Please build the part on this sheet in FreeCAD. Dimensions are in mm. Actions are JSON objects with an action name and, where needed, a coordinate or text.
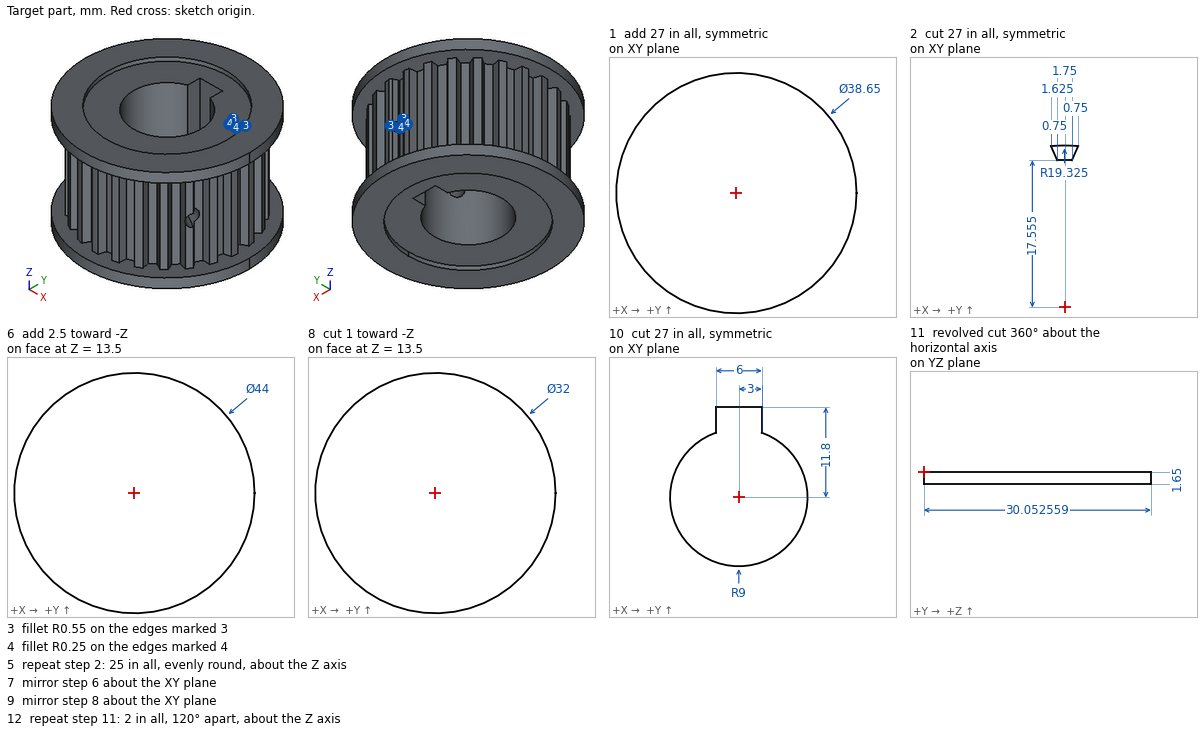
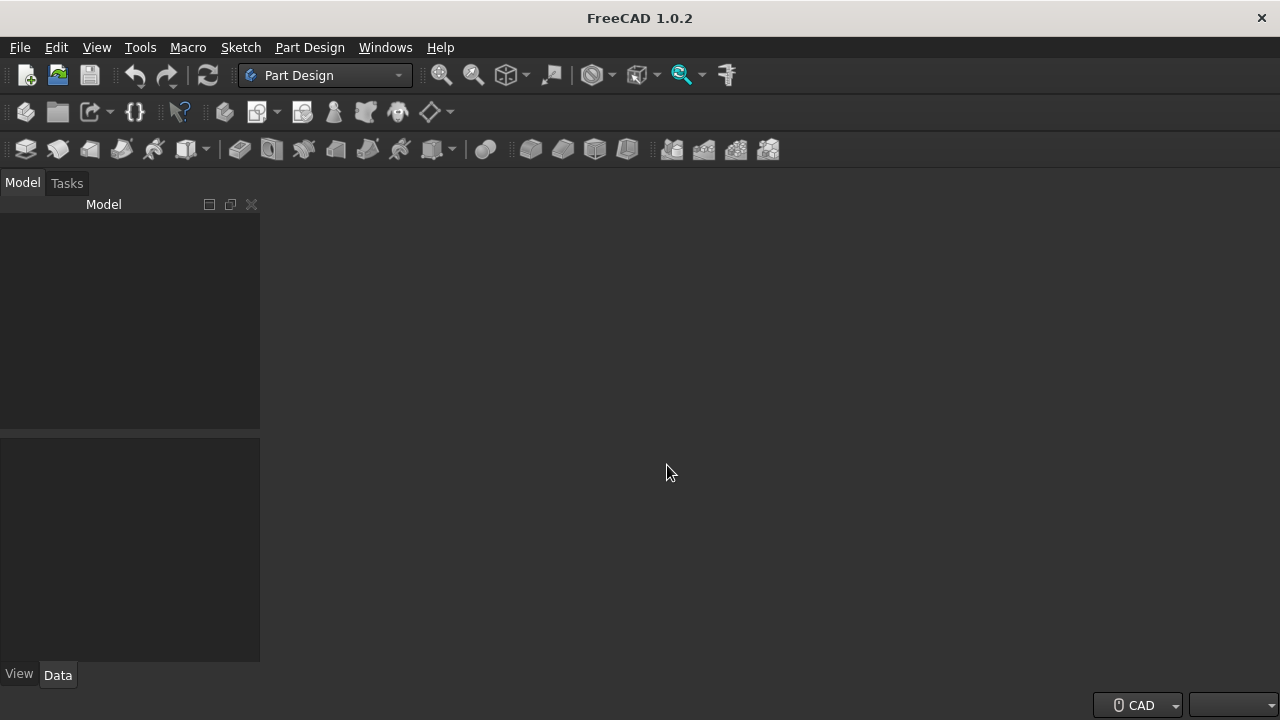
{"action": "left_click", "coordinate": [26, 76]}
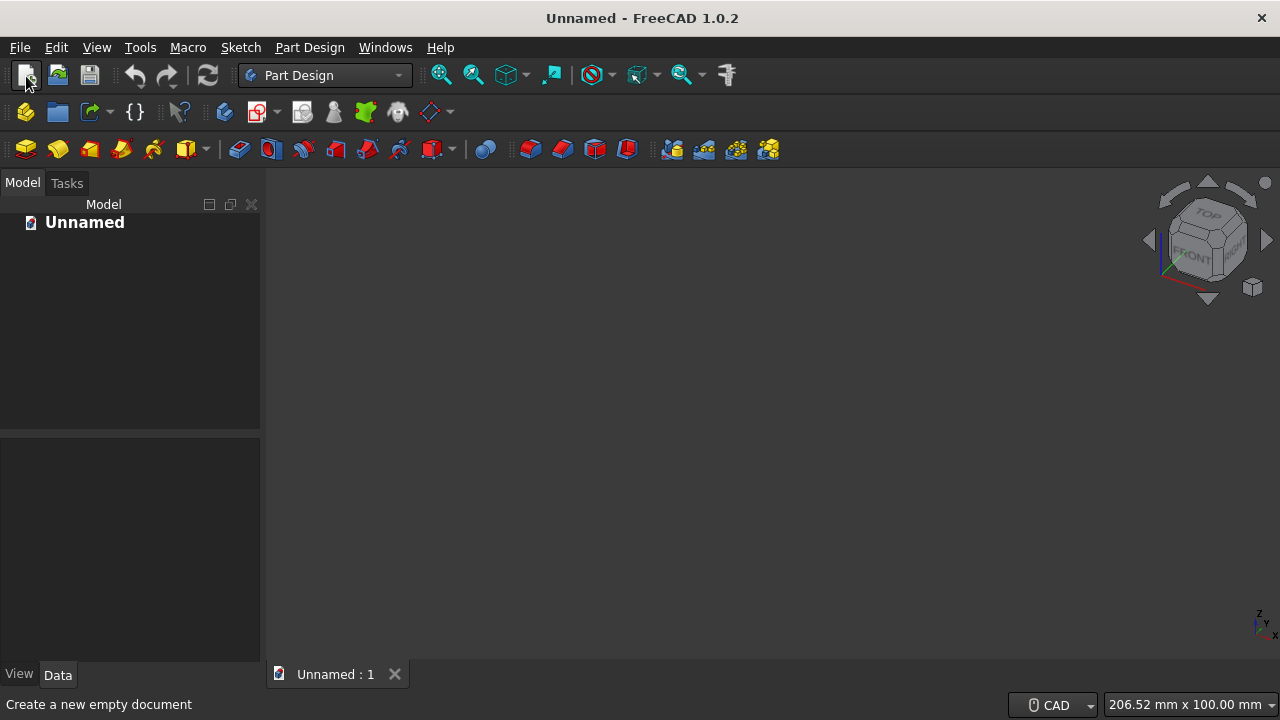
{"action": "left_click", "coordinate": [258, 112]}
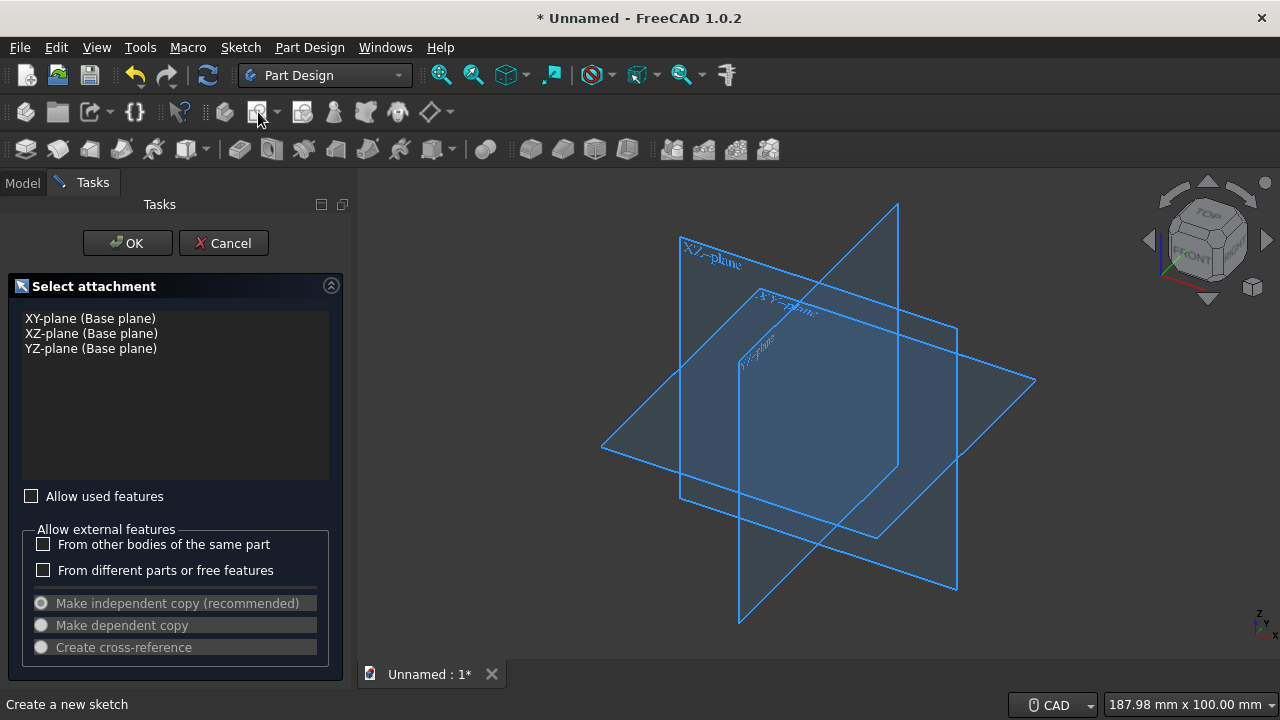
{"action": "left_click", "coordinate": [82, 318]}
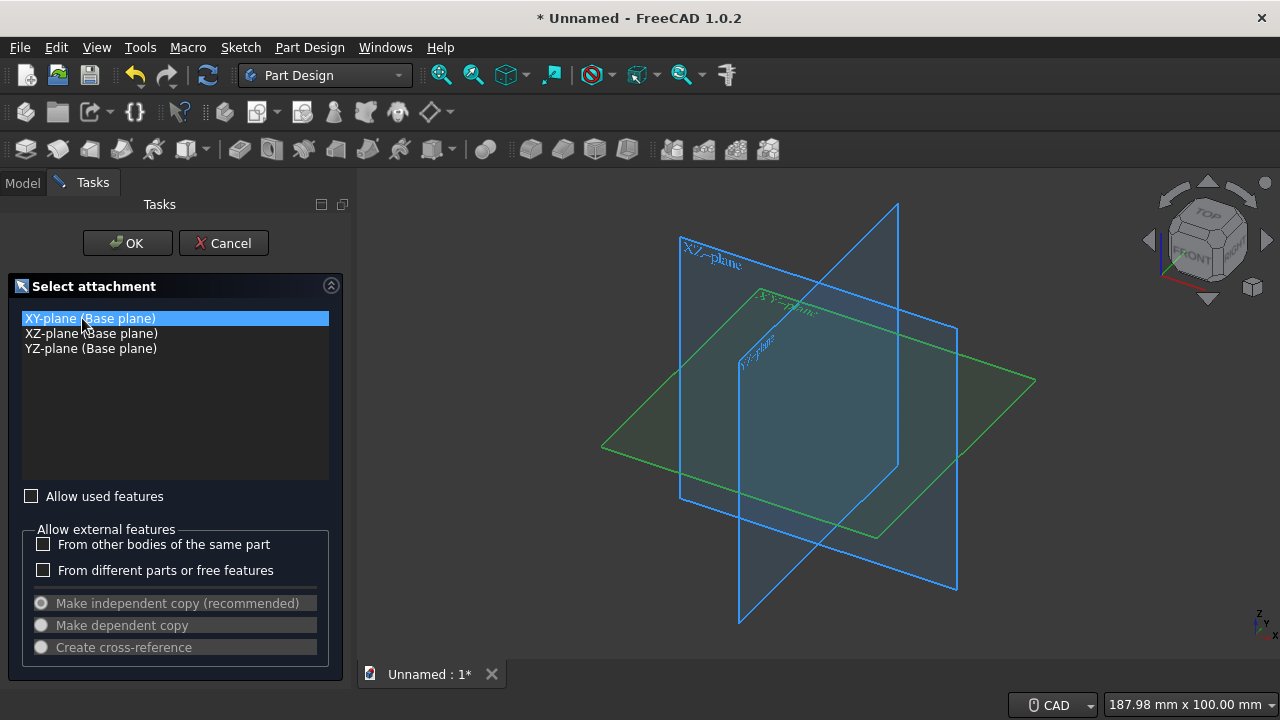
{"action": "left_click", "coordinate": [128, 243]}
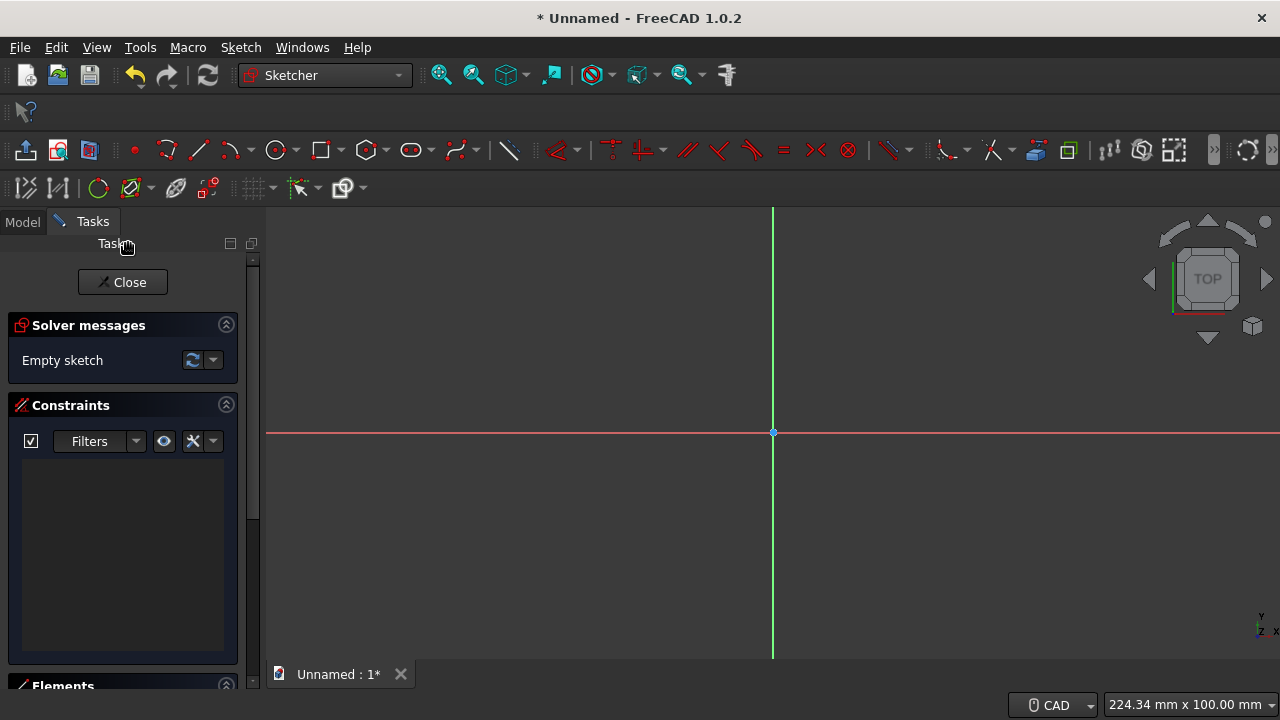
{"action": "scroll", "coordinate": [912, 433], "scroll_direction": "up", "scroll_amount": 2}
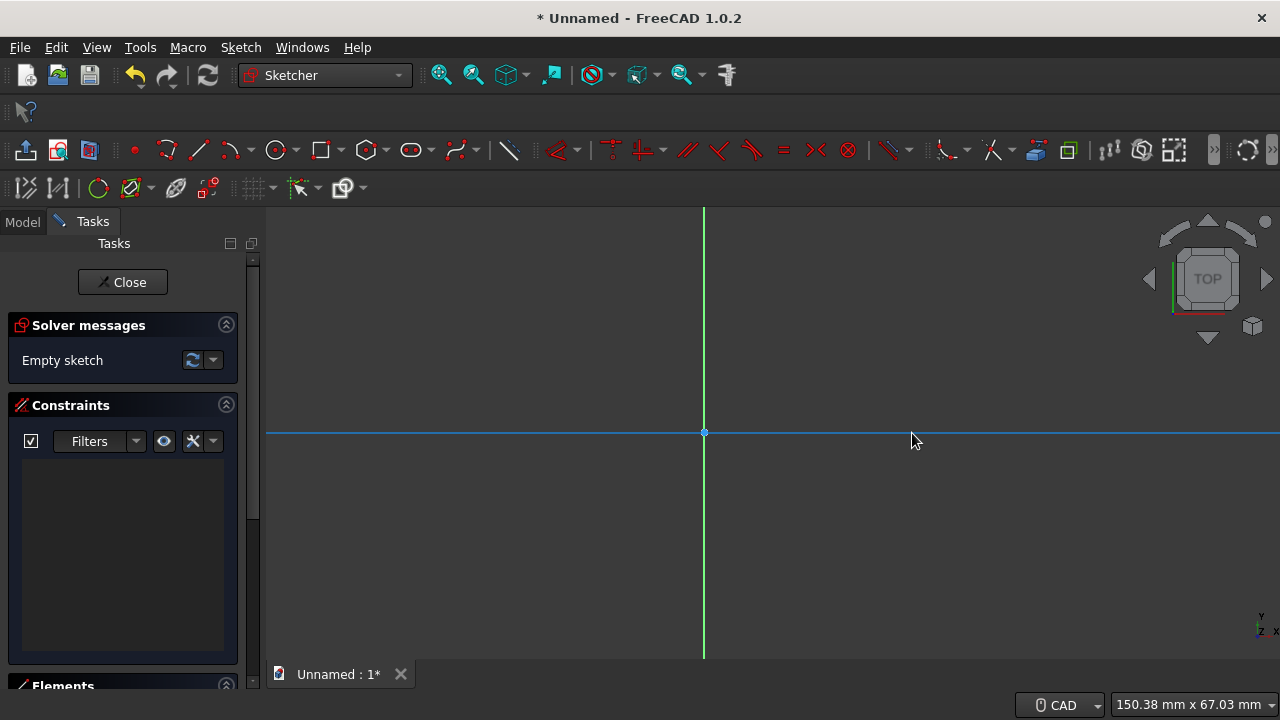
{"action": "left_click", "coordinate": [276, 150]}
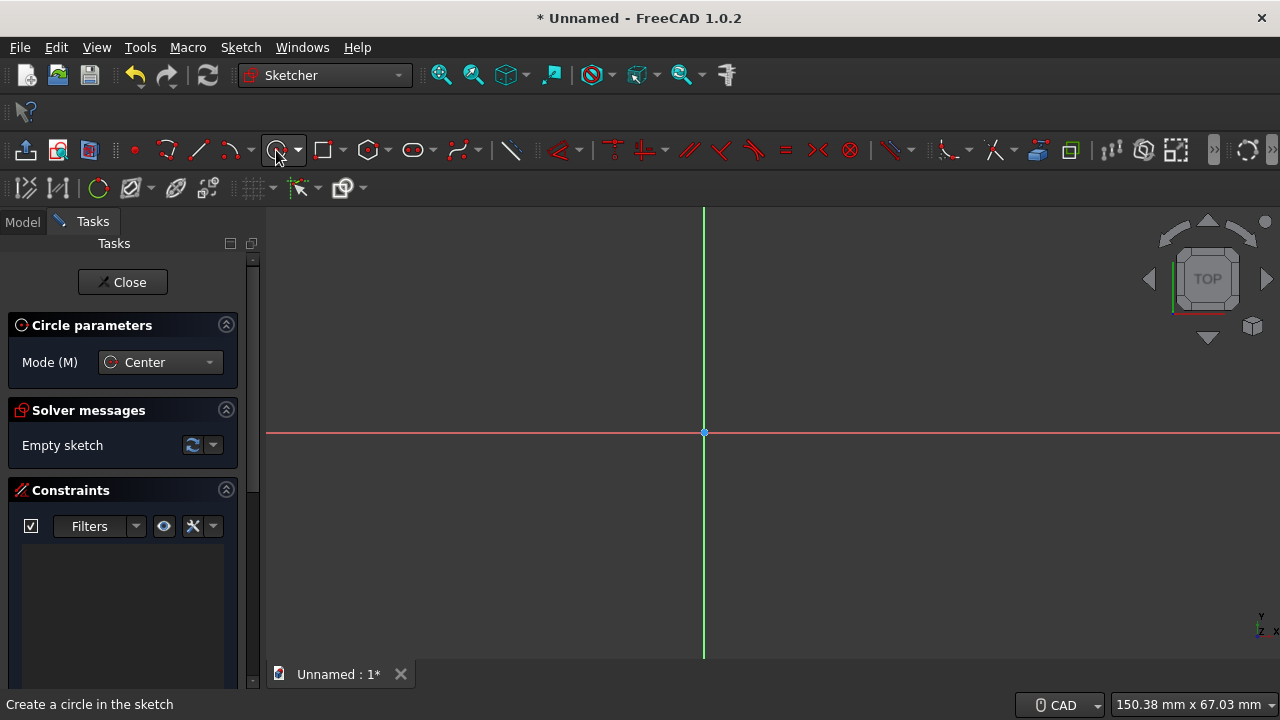
{"action": "left_click", "coordinate": [704, 433]}
{"action": "mouse_move", "coordinate": [796, 341]}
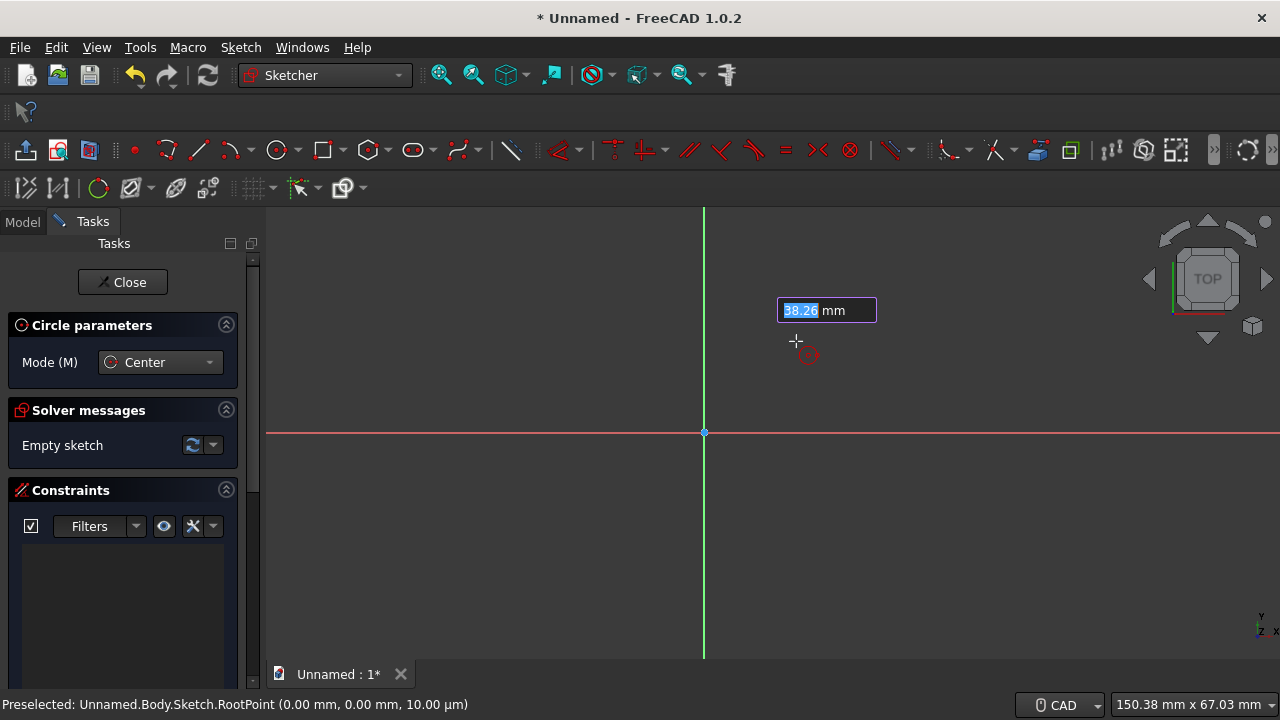
{"action": "type", "text": "38.65"}
{"action": "key", "text": "Return"}
{"action": "key", "text": "Escape"}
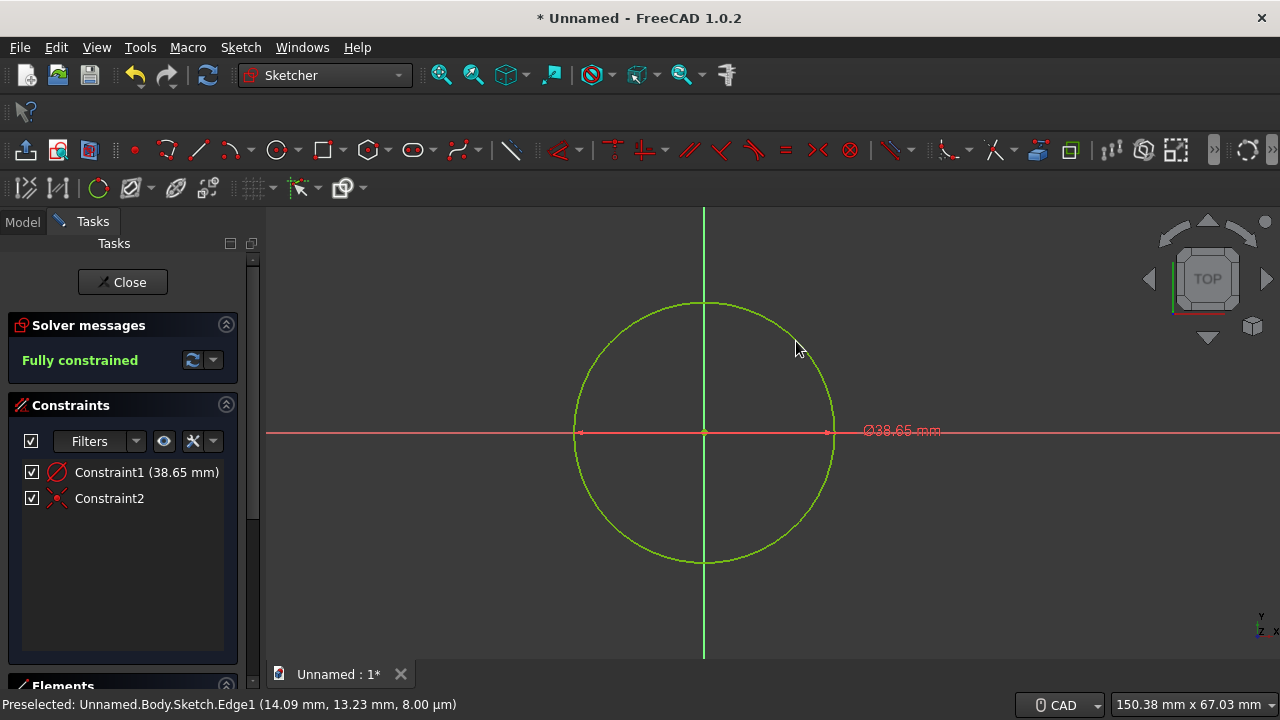
{"action": "left_click", "coordinate": [123, 282]}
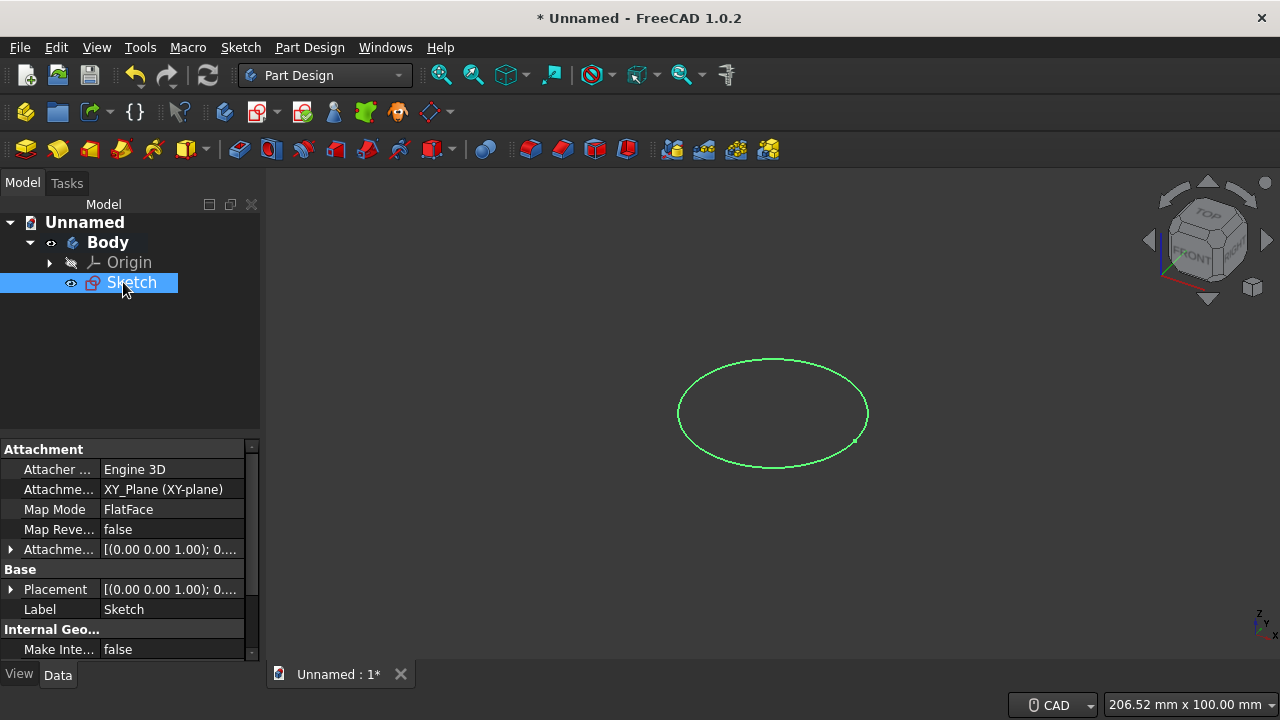
{"action": "left_click", "coordinate": [26, 150]}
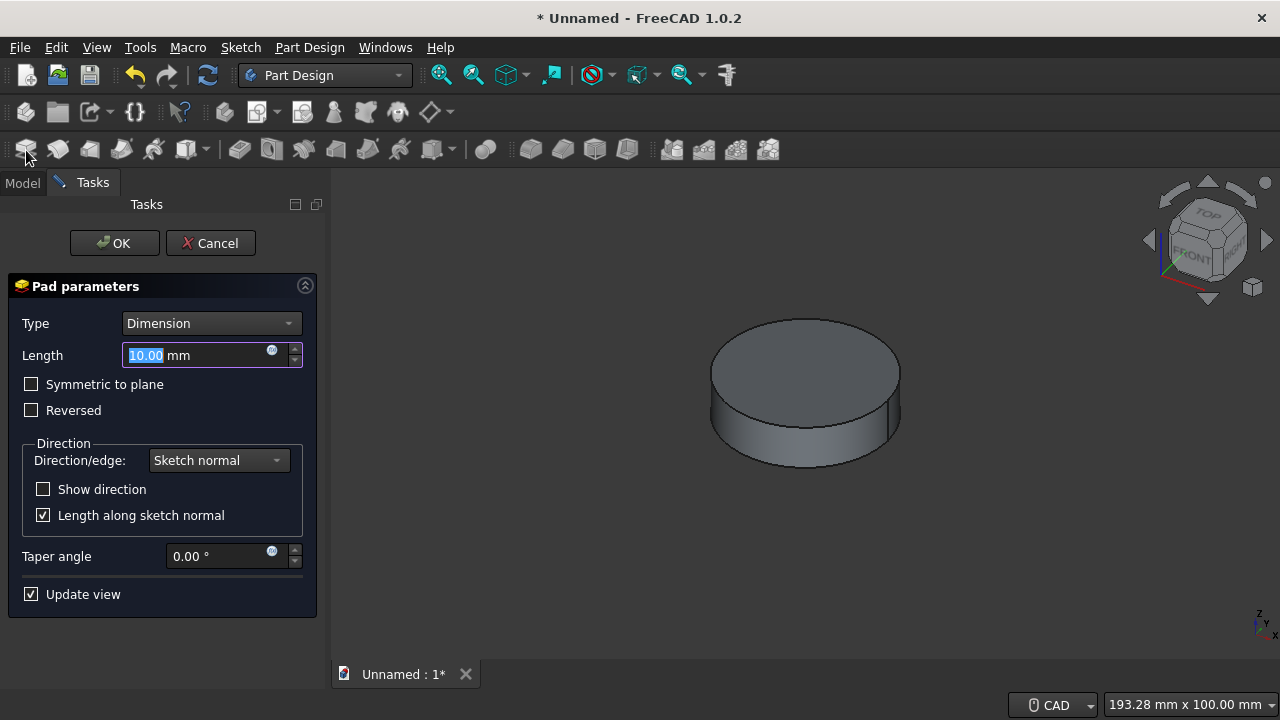
{"action": "type", "text": "27"}
{"action": "key", "text": "Tab"}